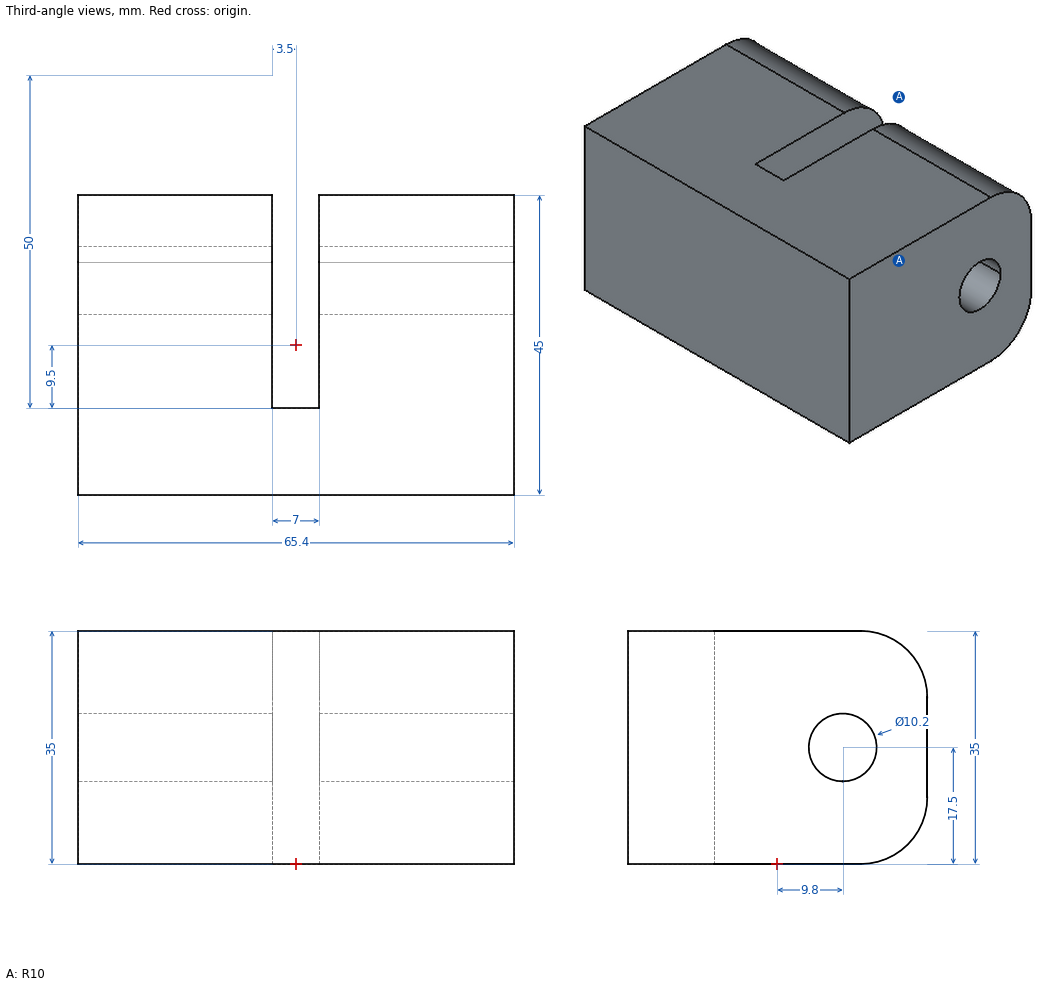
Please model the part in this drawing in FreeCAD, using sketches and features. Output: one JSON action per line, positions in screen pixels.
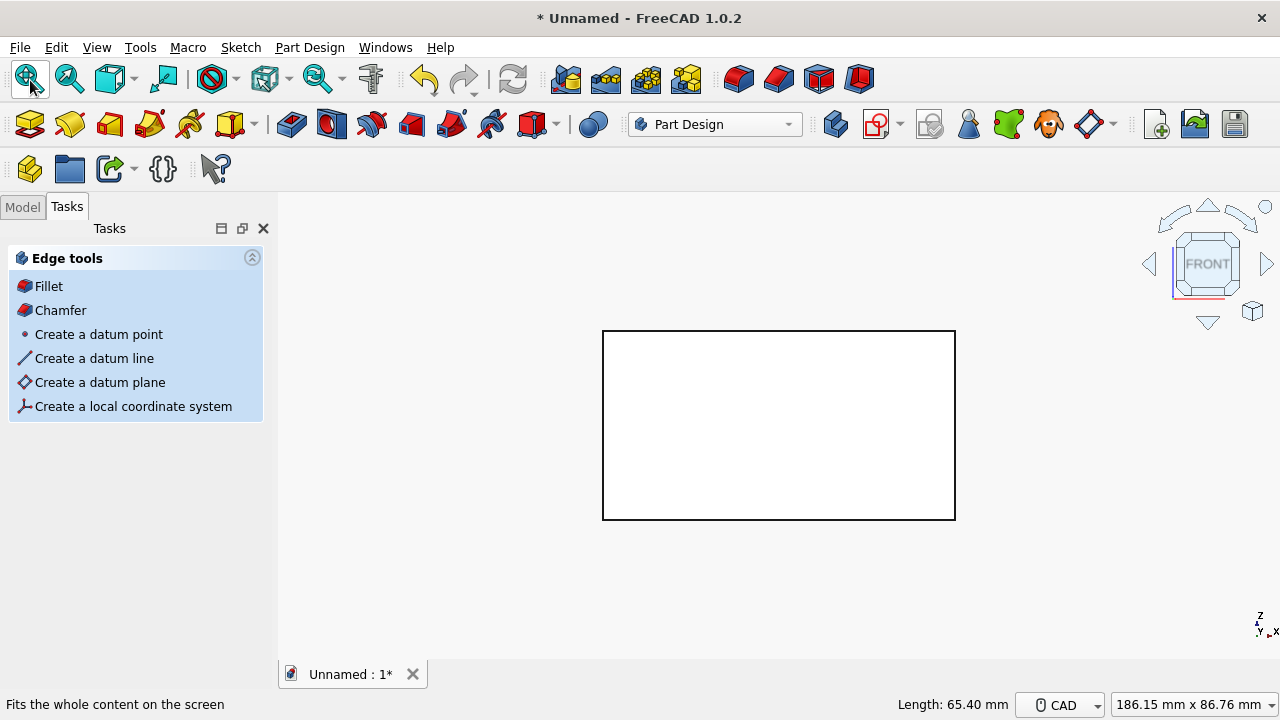
{"action": "key", "text": "3"}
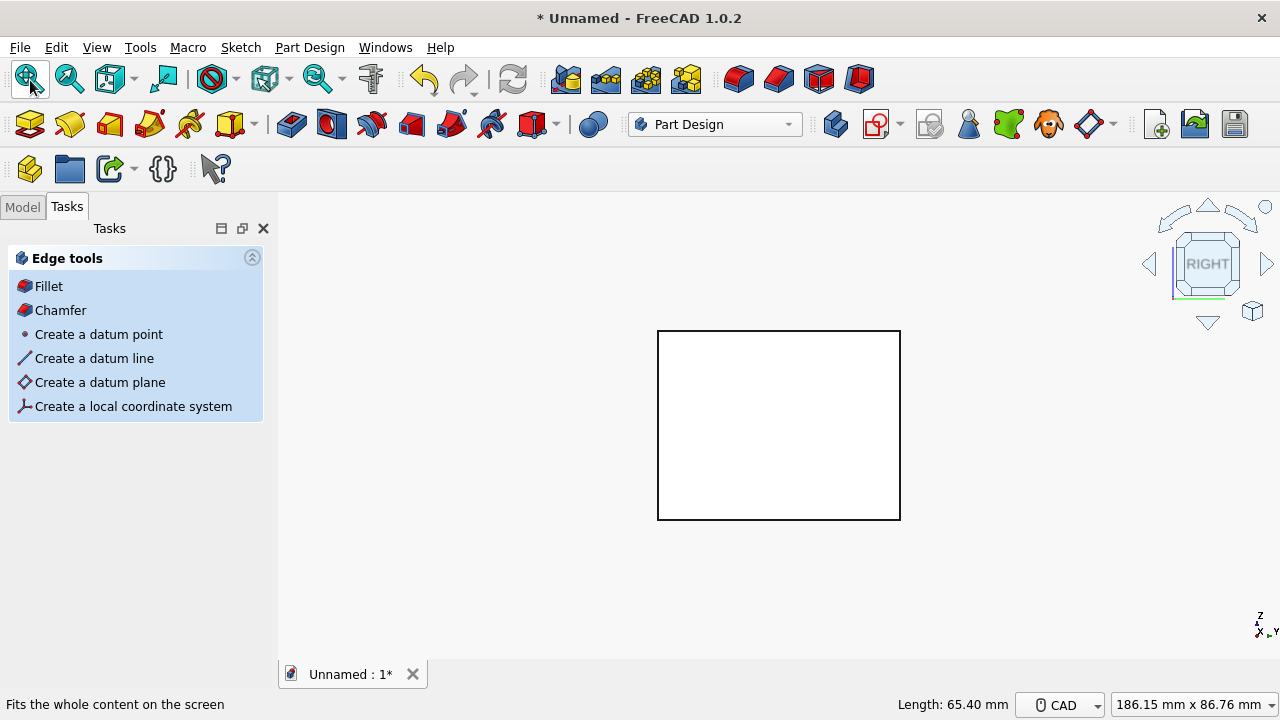
{"action": "left_click", "coordinate": [30, 80]}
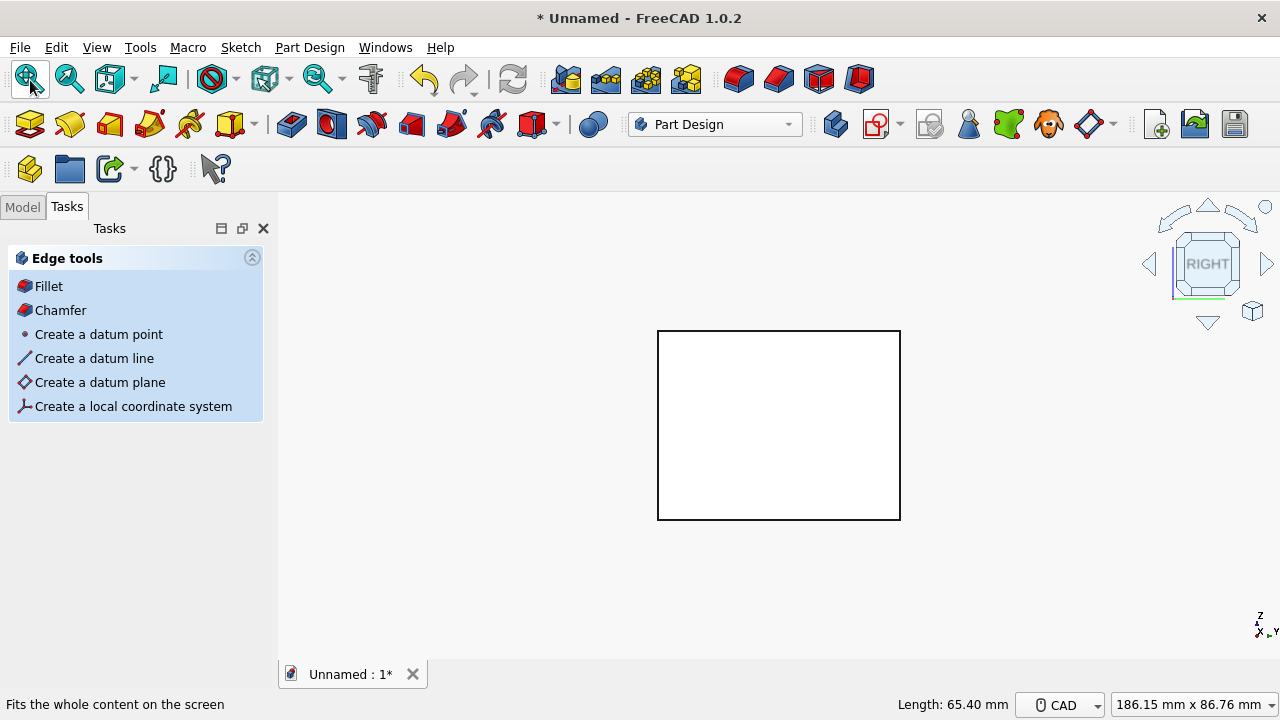
{"action": "key", "text": "5"}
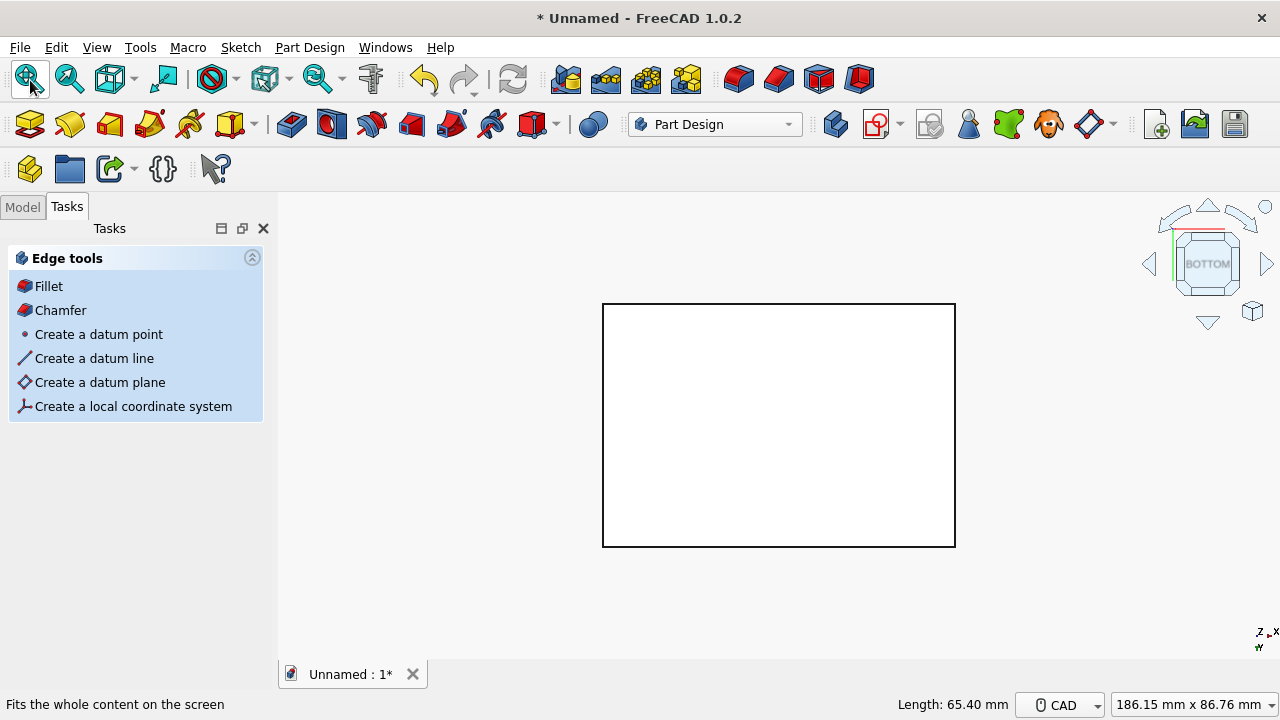
{"action": "left_click", "coordinate": [779, 546], "text": "ctrl"}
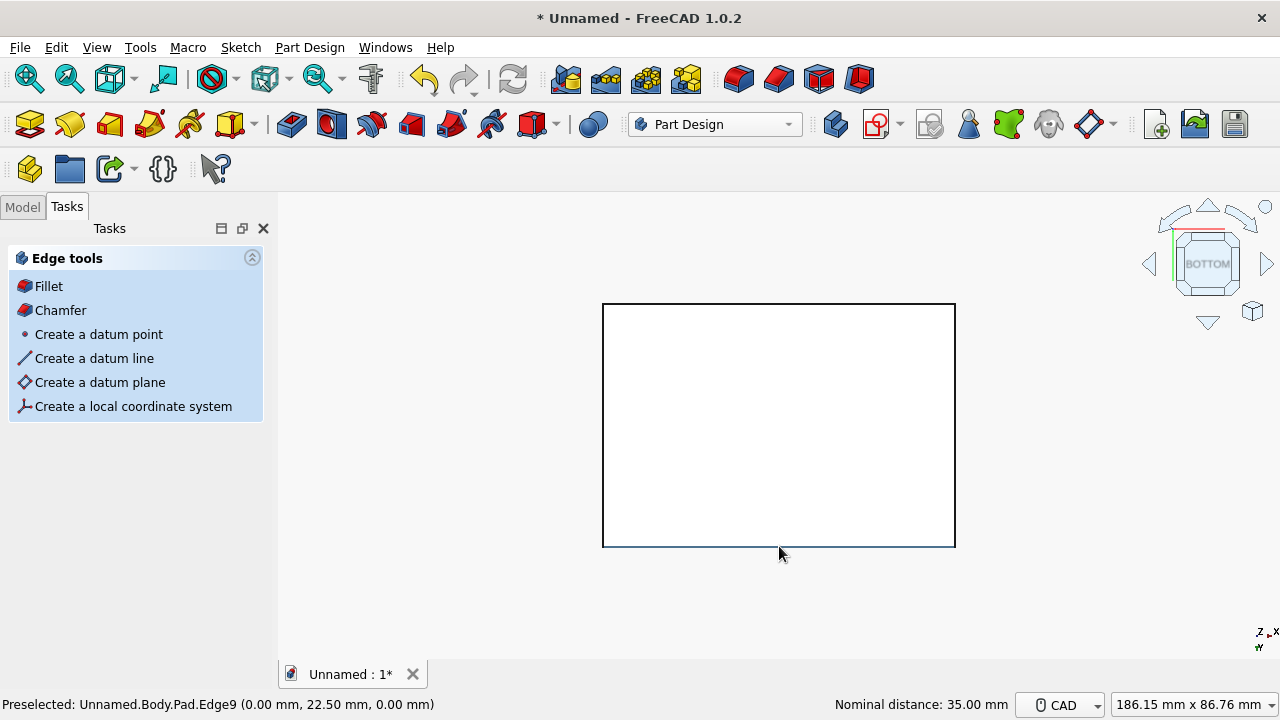
{"action": "left_click", "coordinate": [740, 80]}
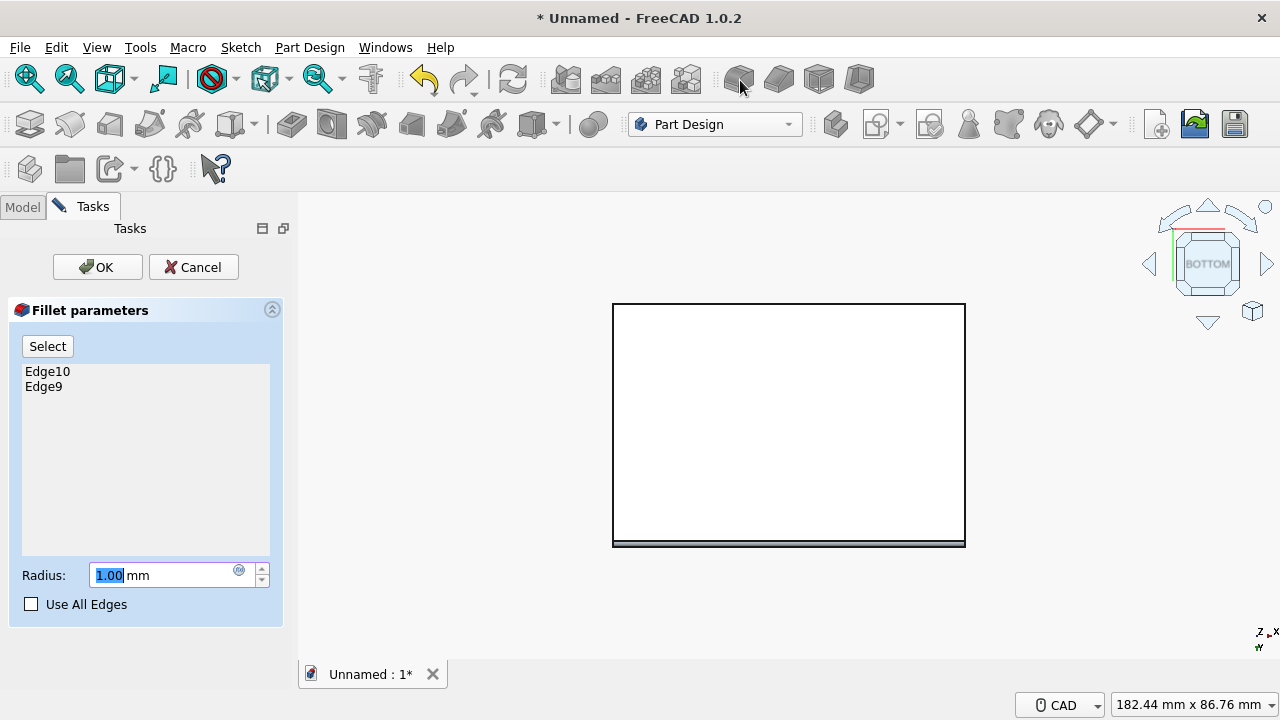
{"action": "type", "text": "10"}
{"action": "key", "text": "Tab"}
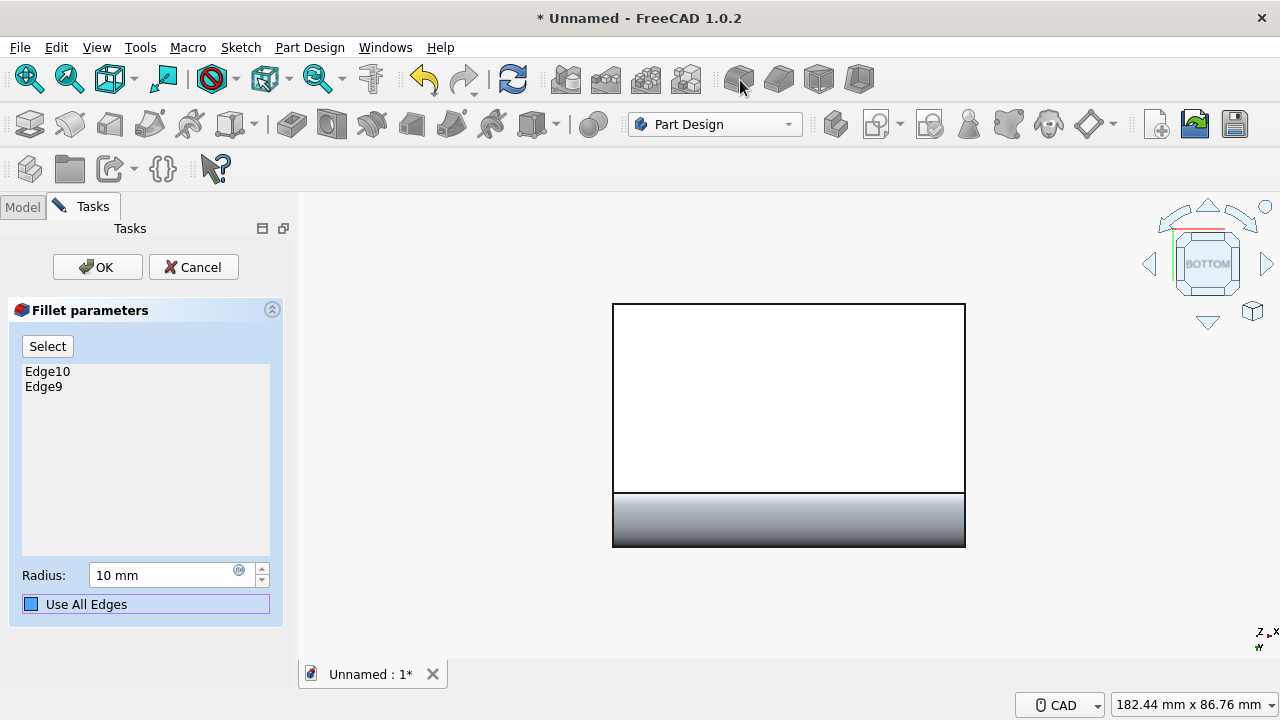
{"action": "left_click", "coordinate": [98, 267]}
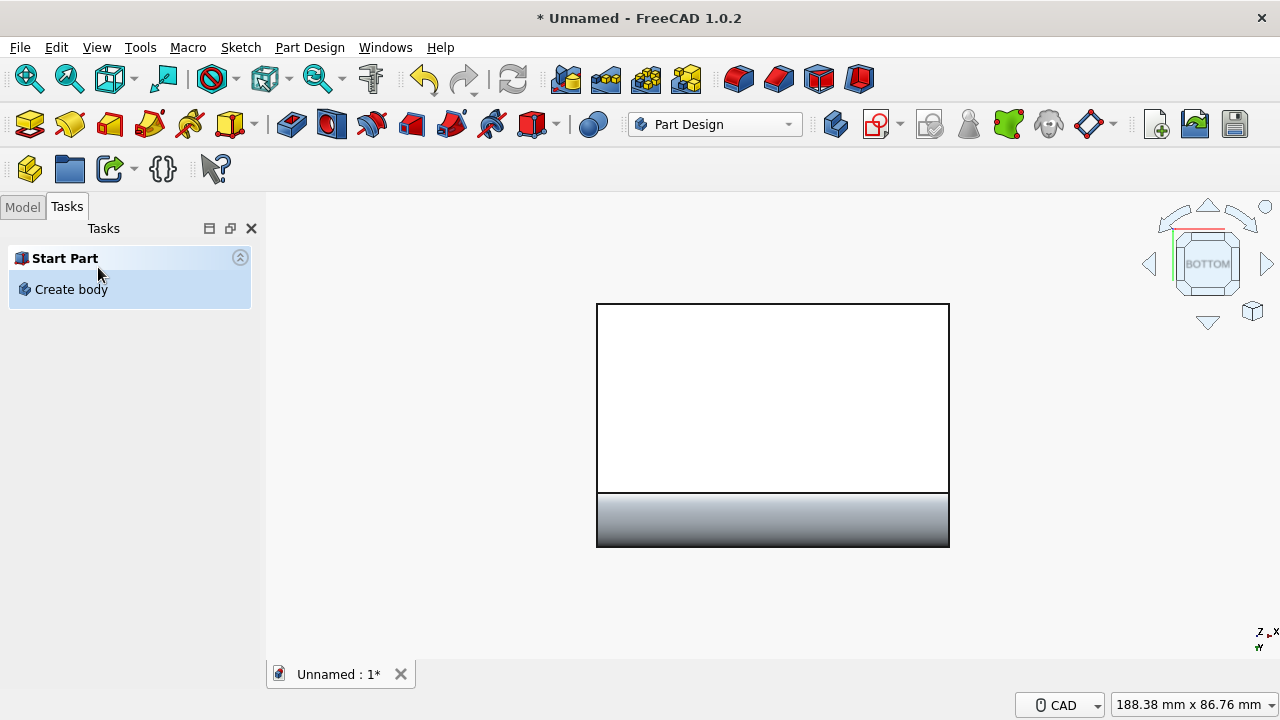
{"action": "key", "text": "0"}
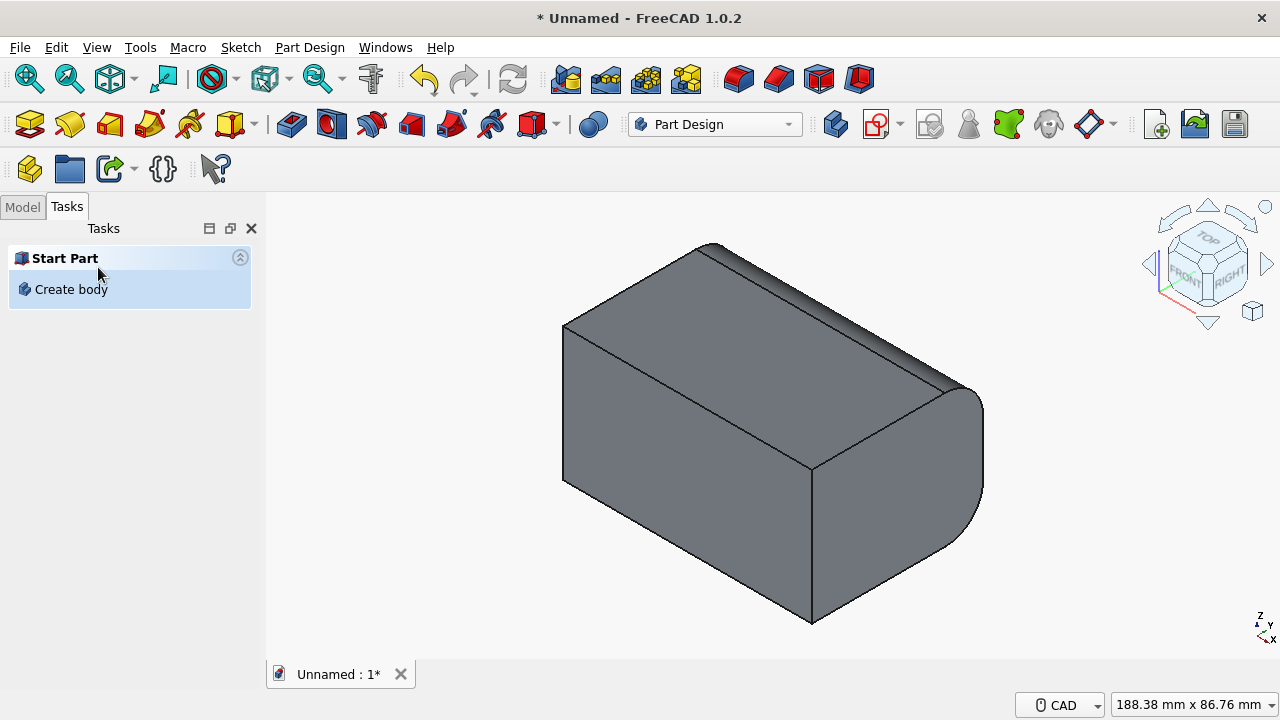
{"action": "left_click", "coordinate": [897, 496]}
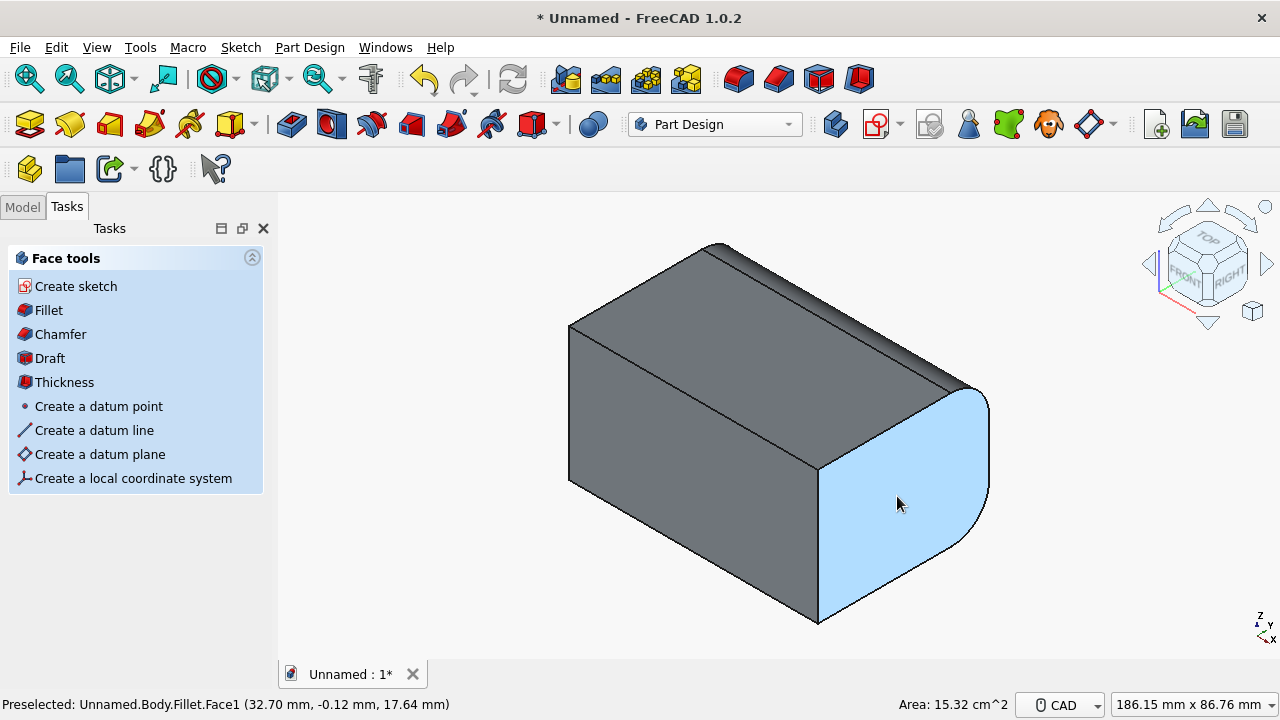
{"action": "left_click", "coordinate": [876, 124]}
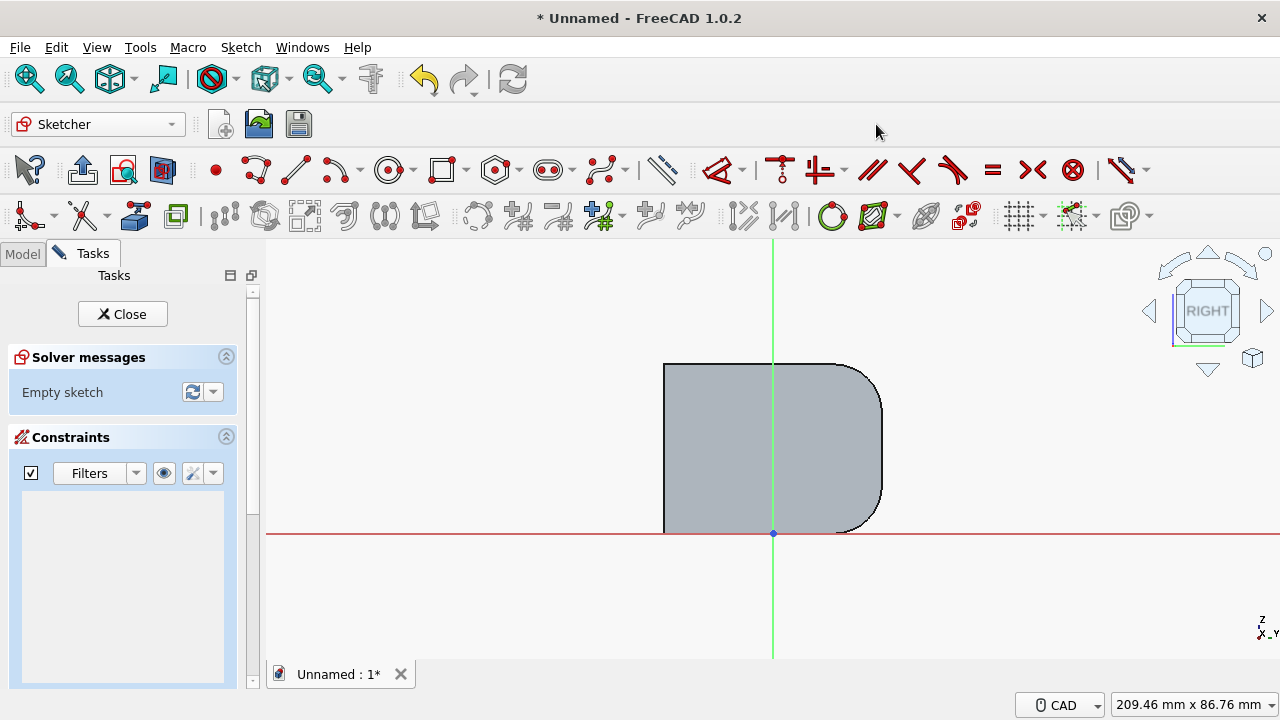
{"action": "scroll", "coordinate": [894, 504], "scroll_direction": "up", "scroll_amount": 4}